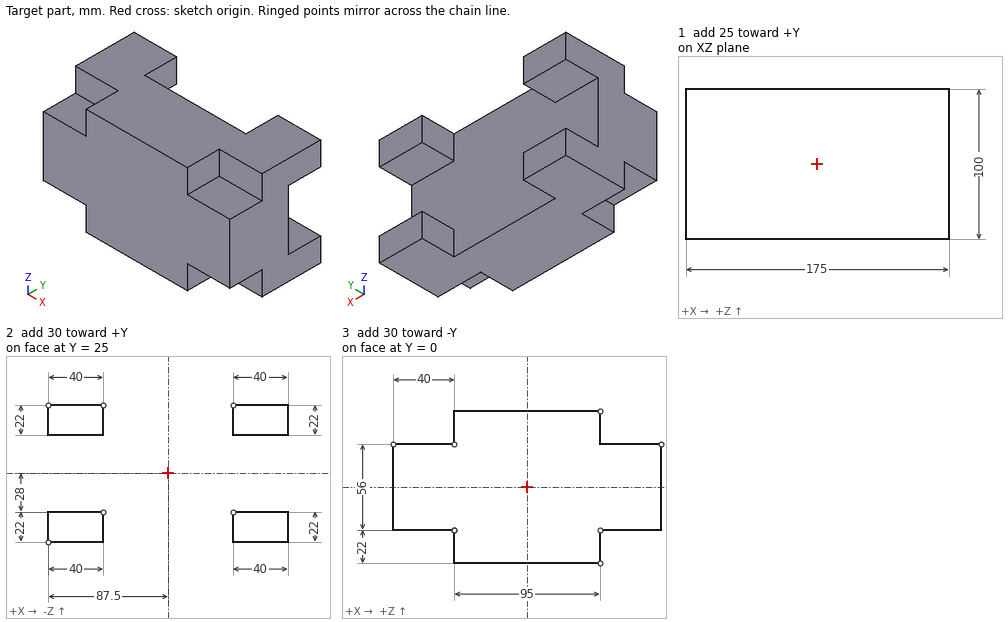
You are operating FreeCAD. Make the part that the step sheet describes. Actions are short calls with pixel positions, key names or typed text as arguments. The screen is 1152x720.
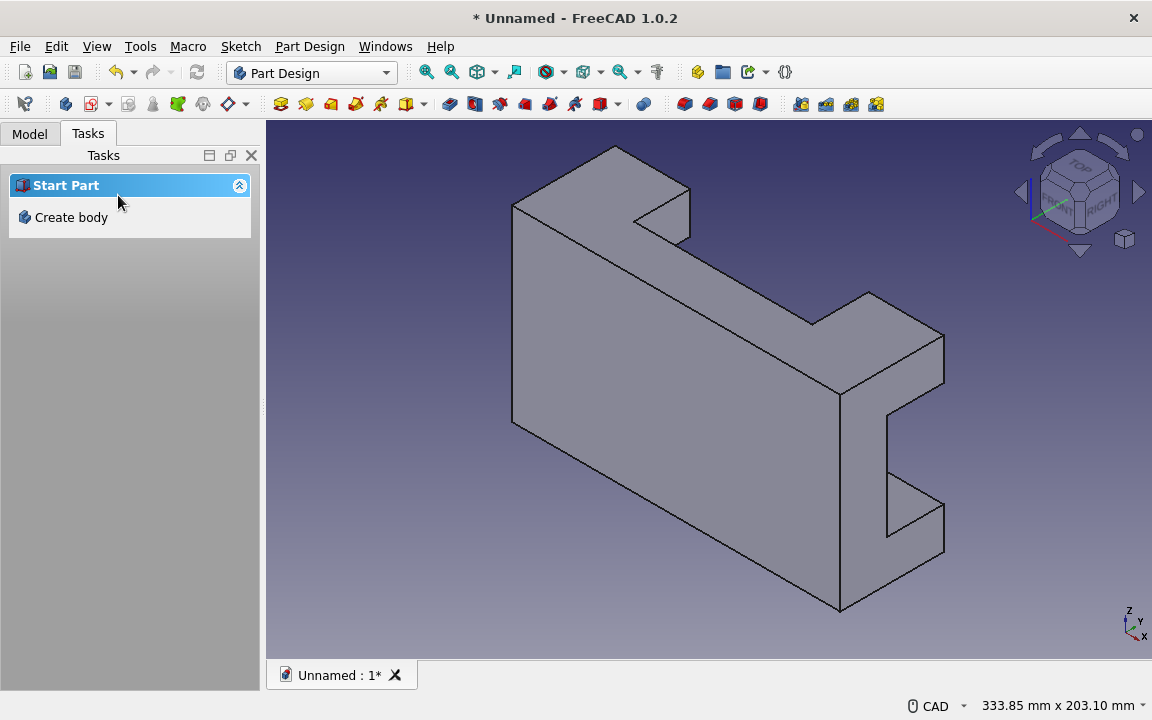
click(723, 435)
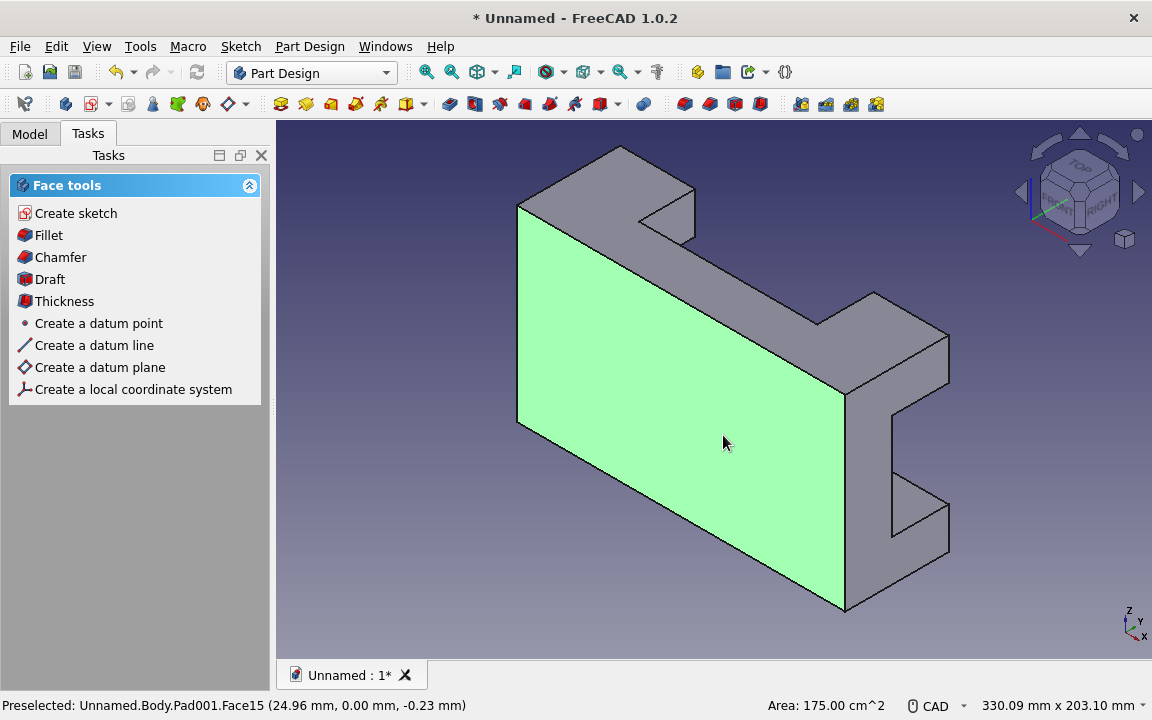
click(90, 104)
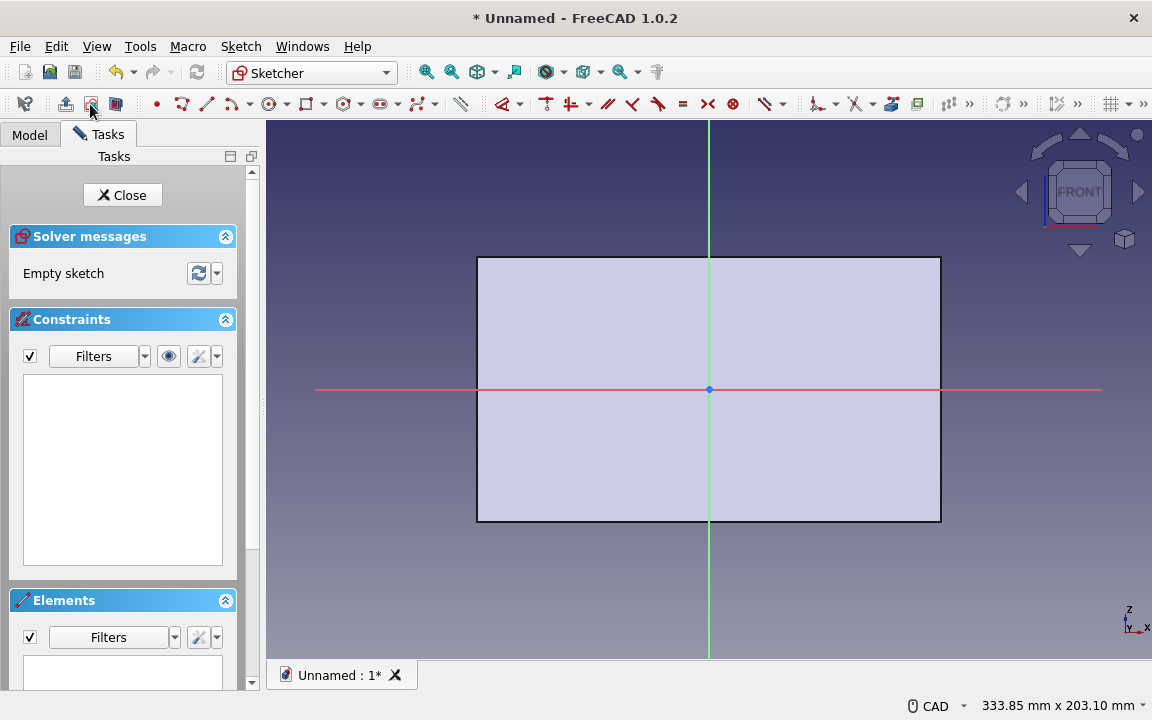
click(182, 104)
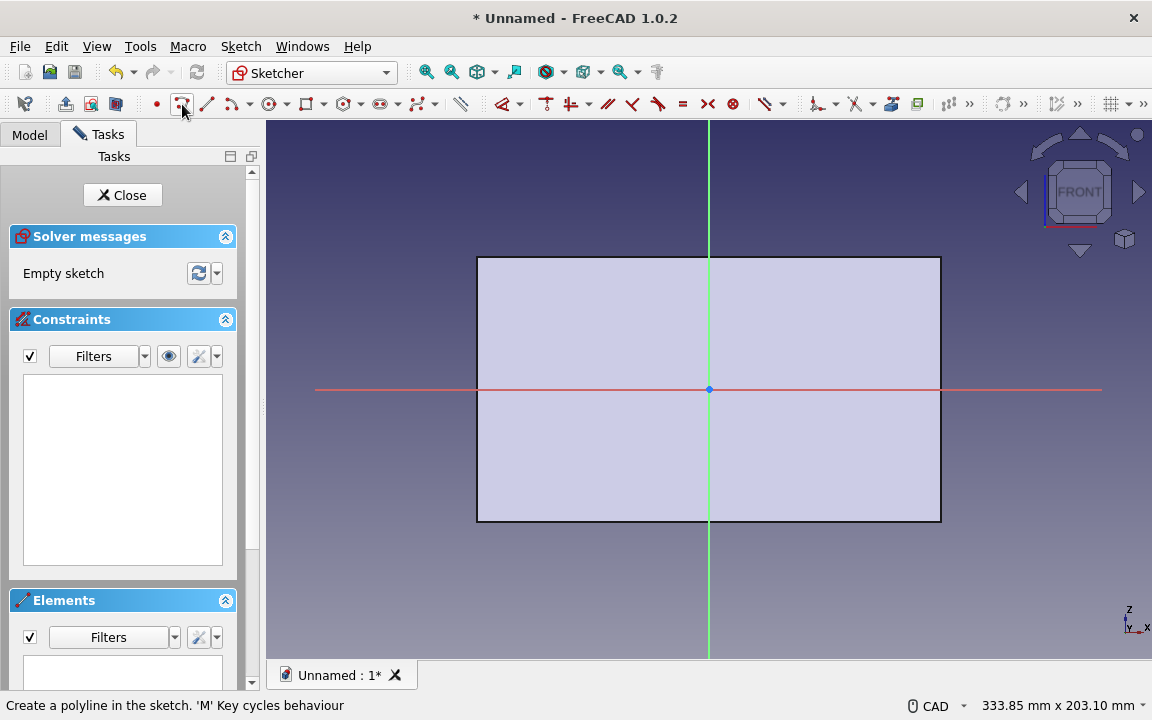
click(583, 315)
click(477, 315)
click(477, 464)
click(583, 464)
click(583, 522)
click(835, 522)
click(835, 464)
click(941, 464)
click(941, 315)
click(835, 315)
click(835, 257)
click(583, 257)
click(583, 316)
key(Escape)
key(Escape)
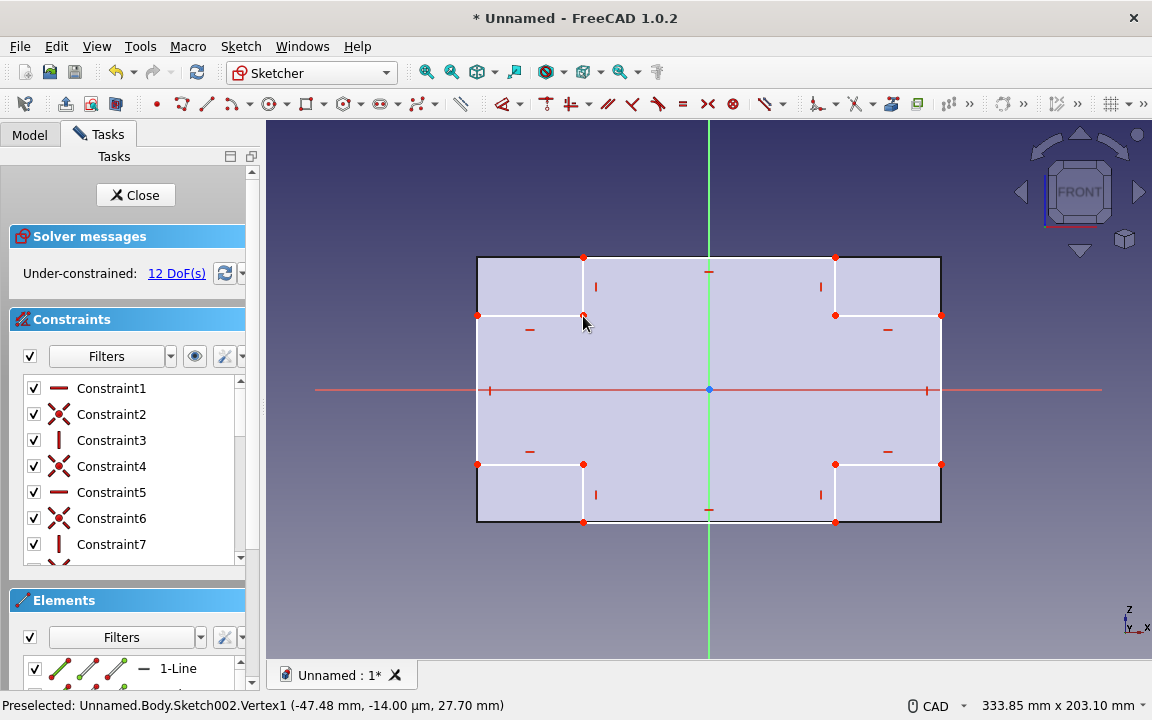
click(583, 316)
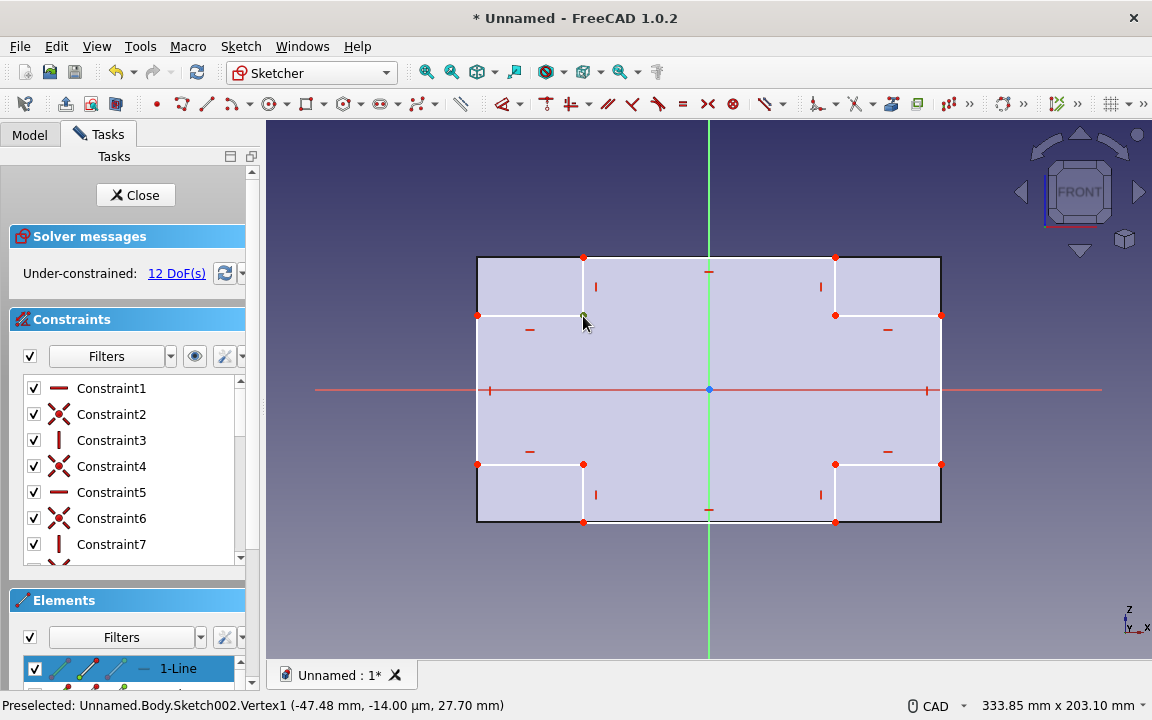
click(583, 465)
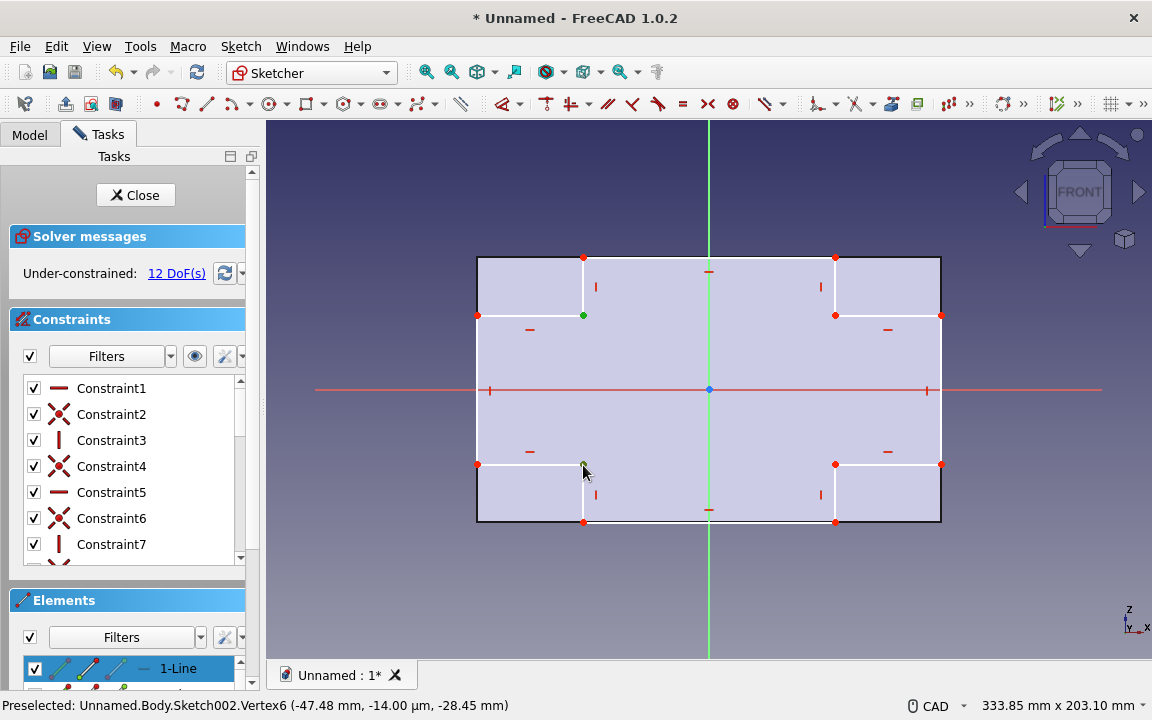
click(344, 390)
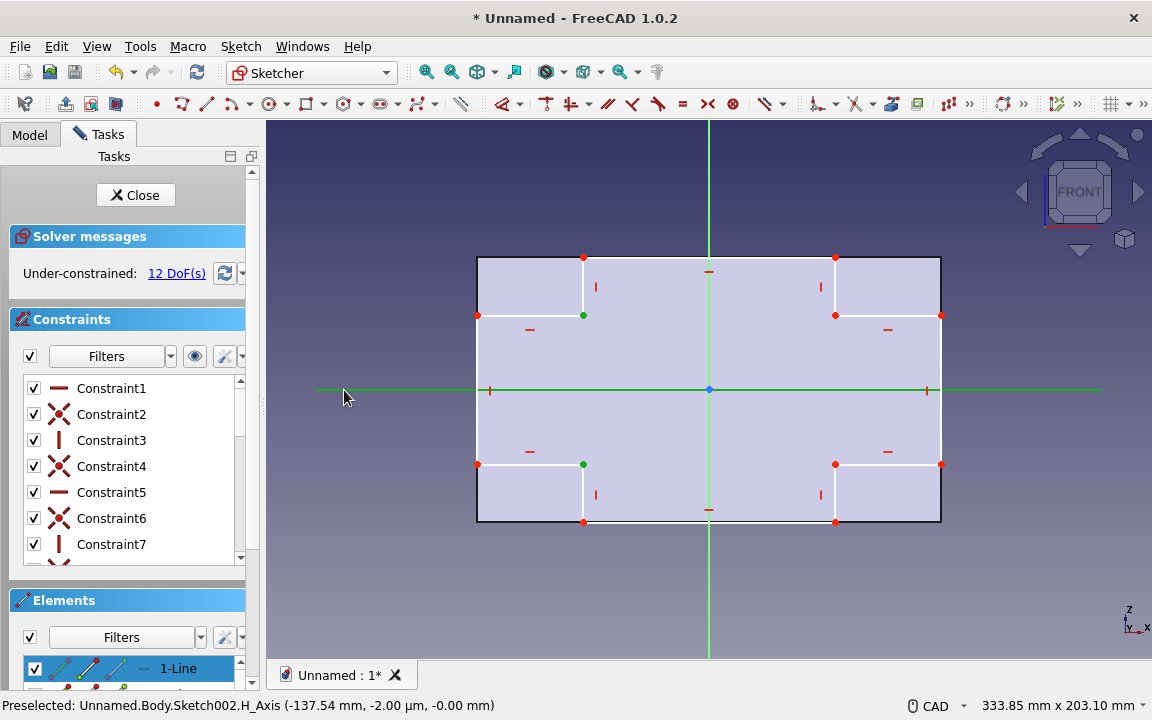
click(708, 104)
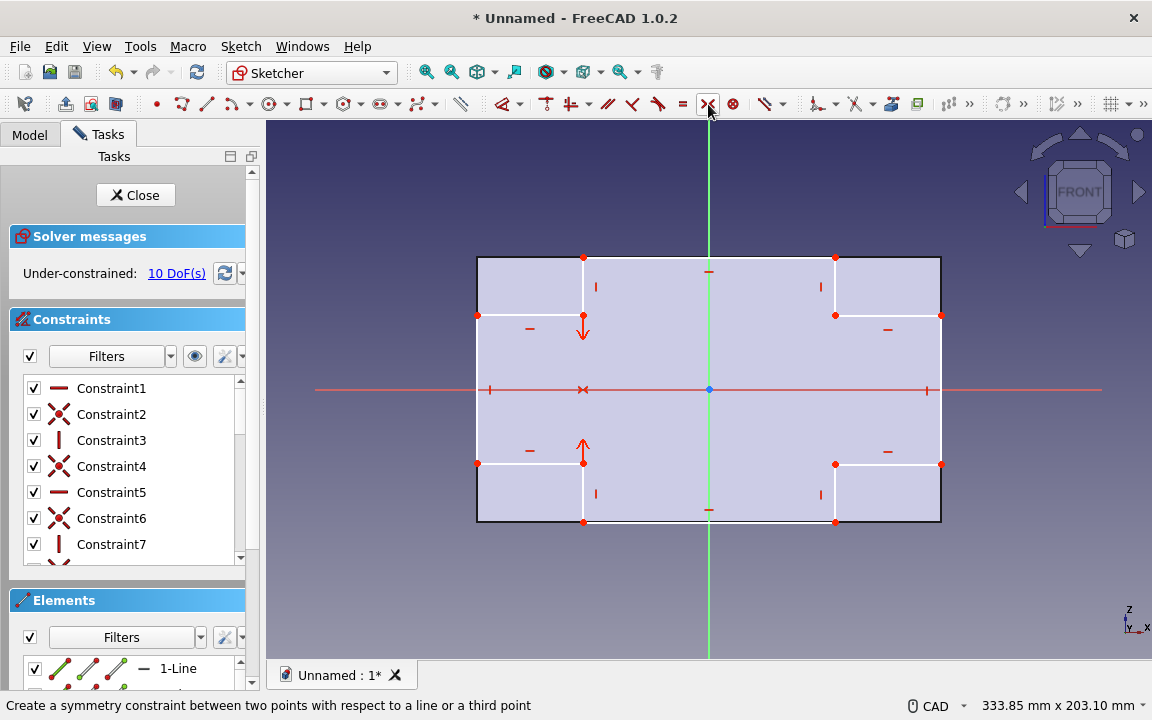
click(583, 464)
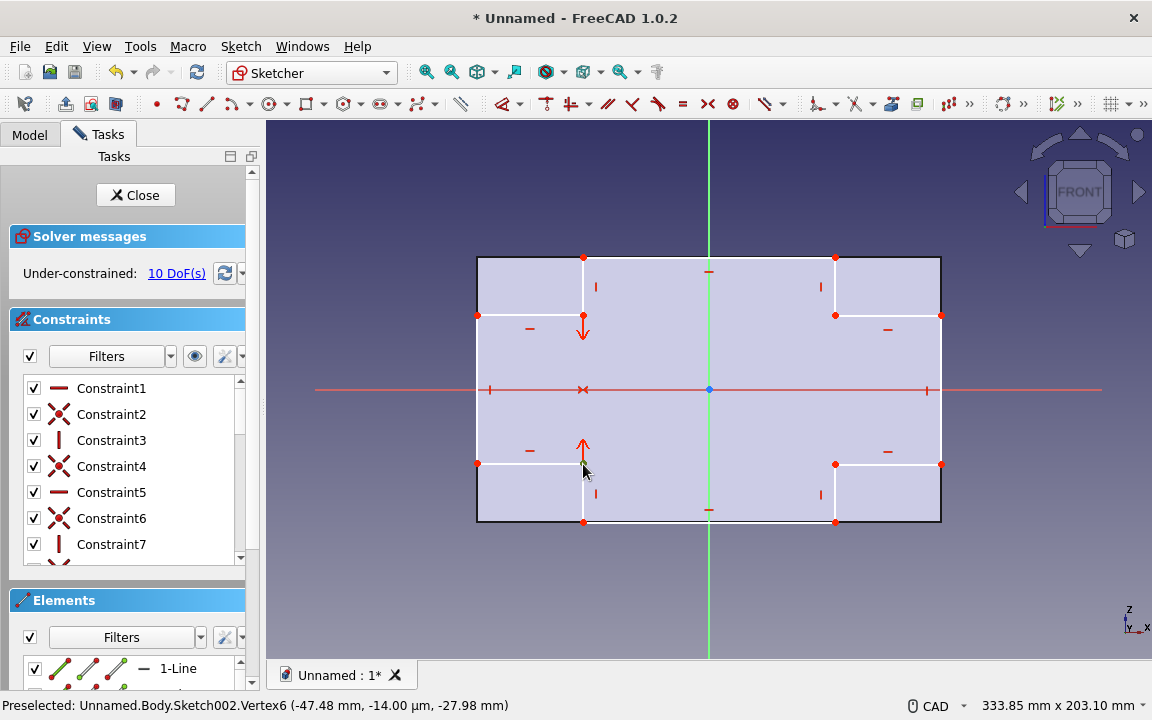
click(835, 465)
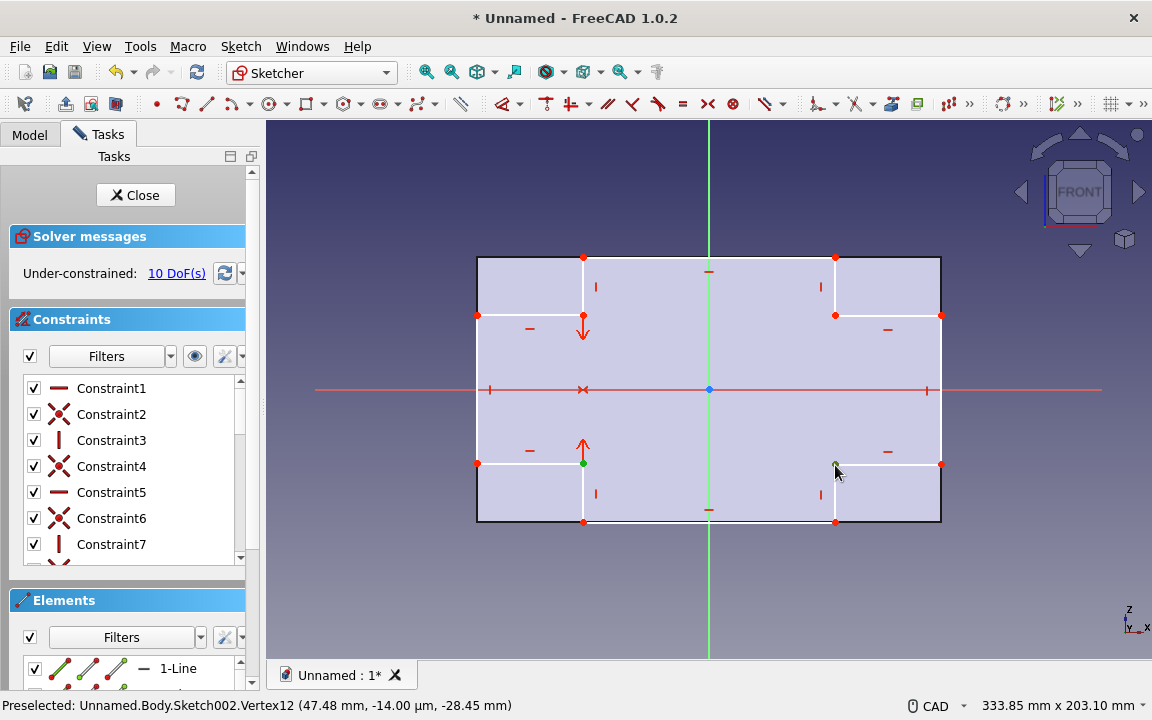
click(709, 596)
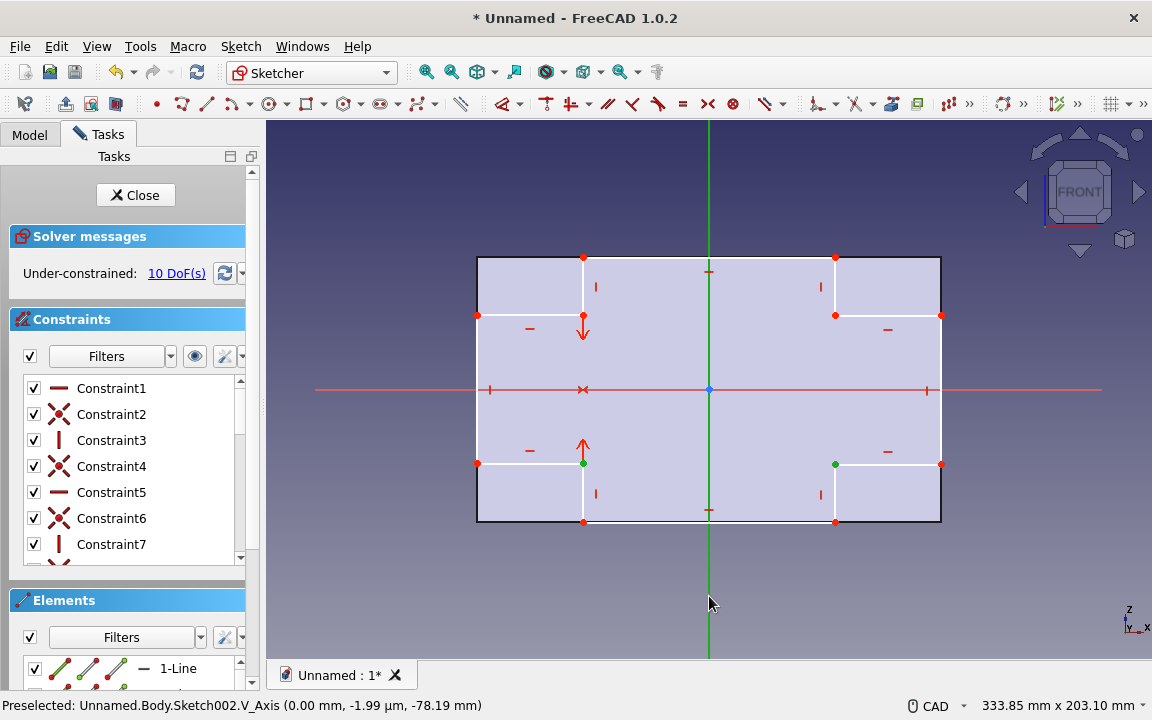
click(708, 104)